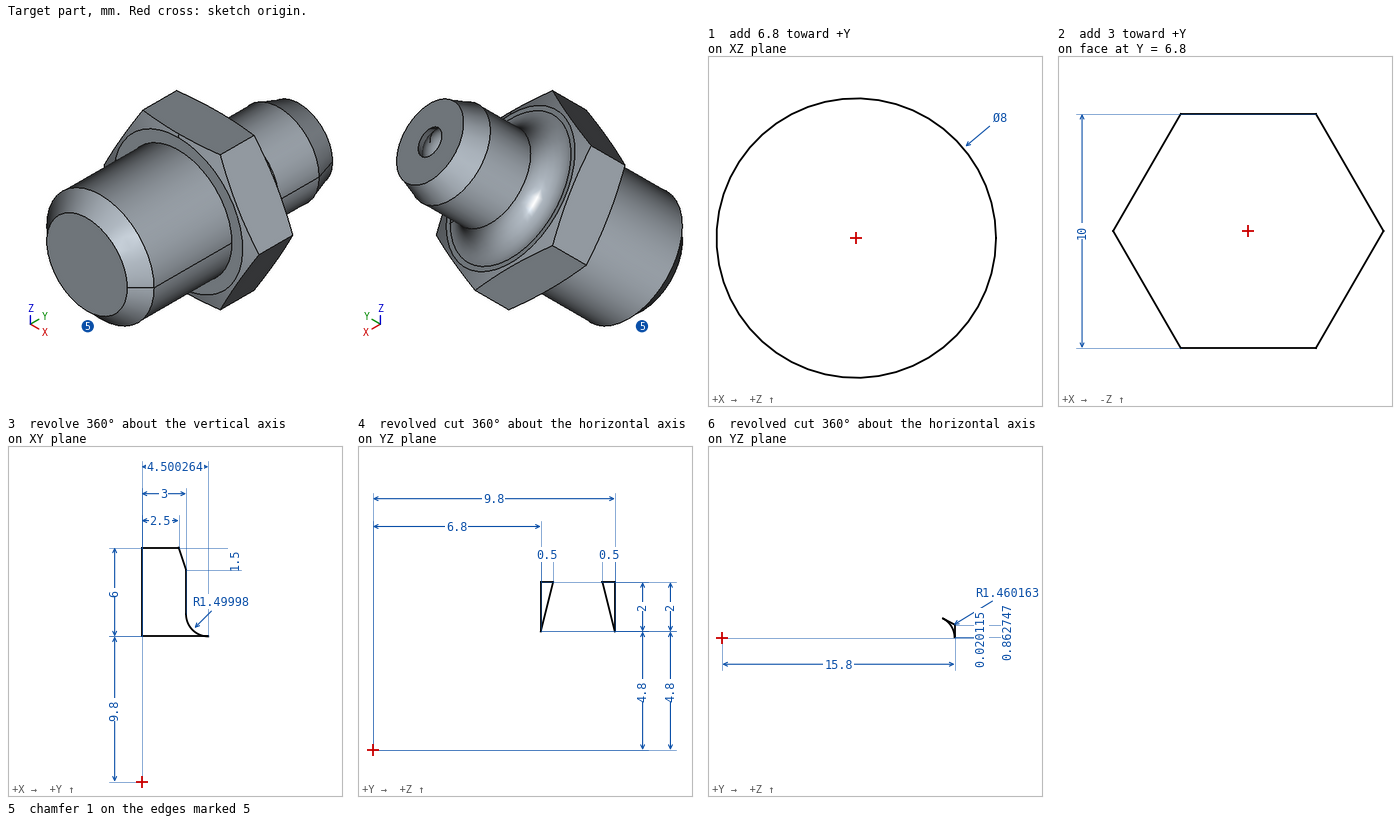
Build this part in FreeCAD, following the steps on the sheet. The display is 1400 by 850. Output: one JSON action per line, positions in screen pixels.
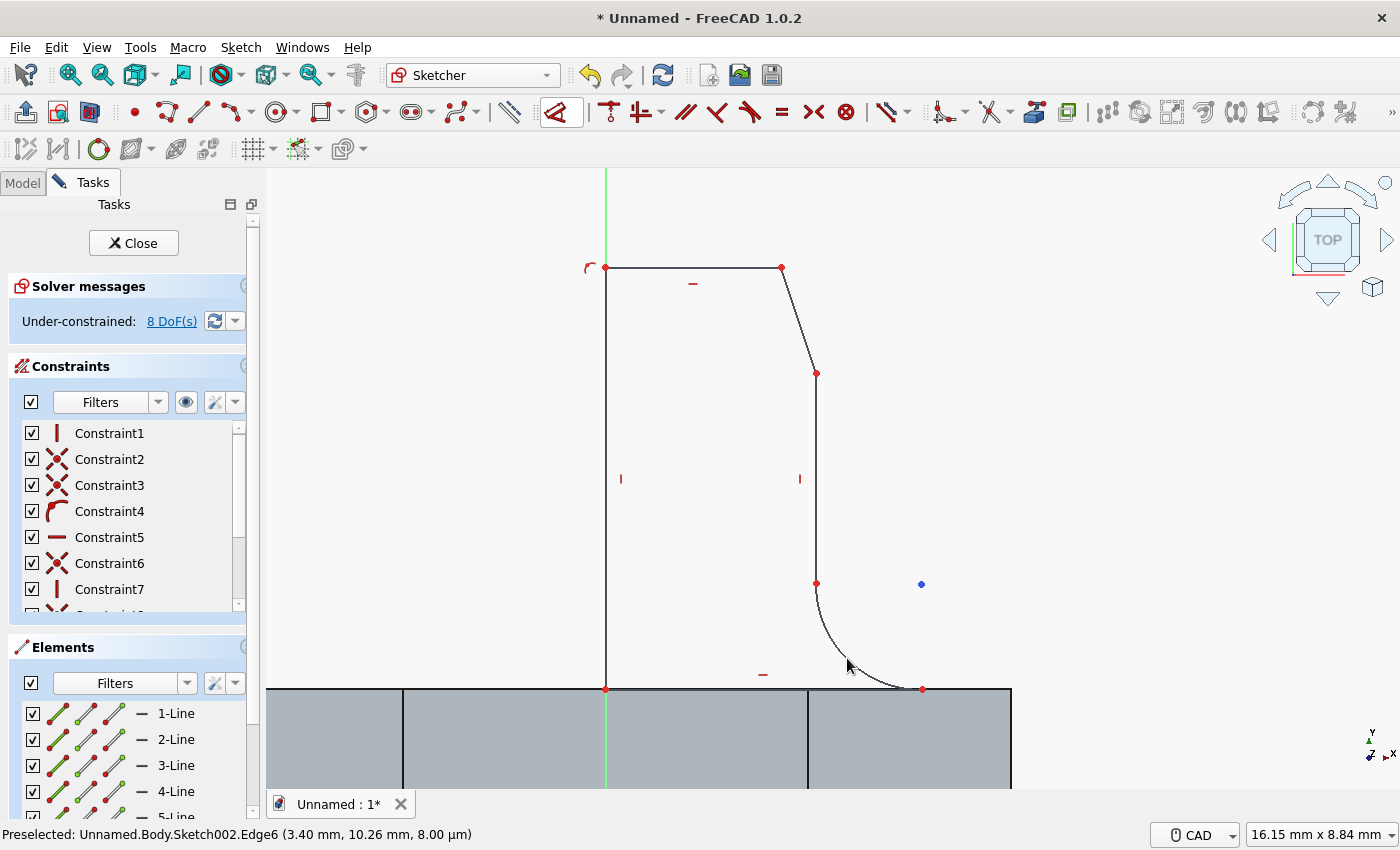
{"action": "left_click", "coordinate": [816, 521]}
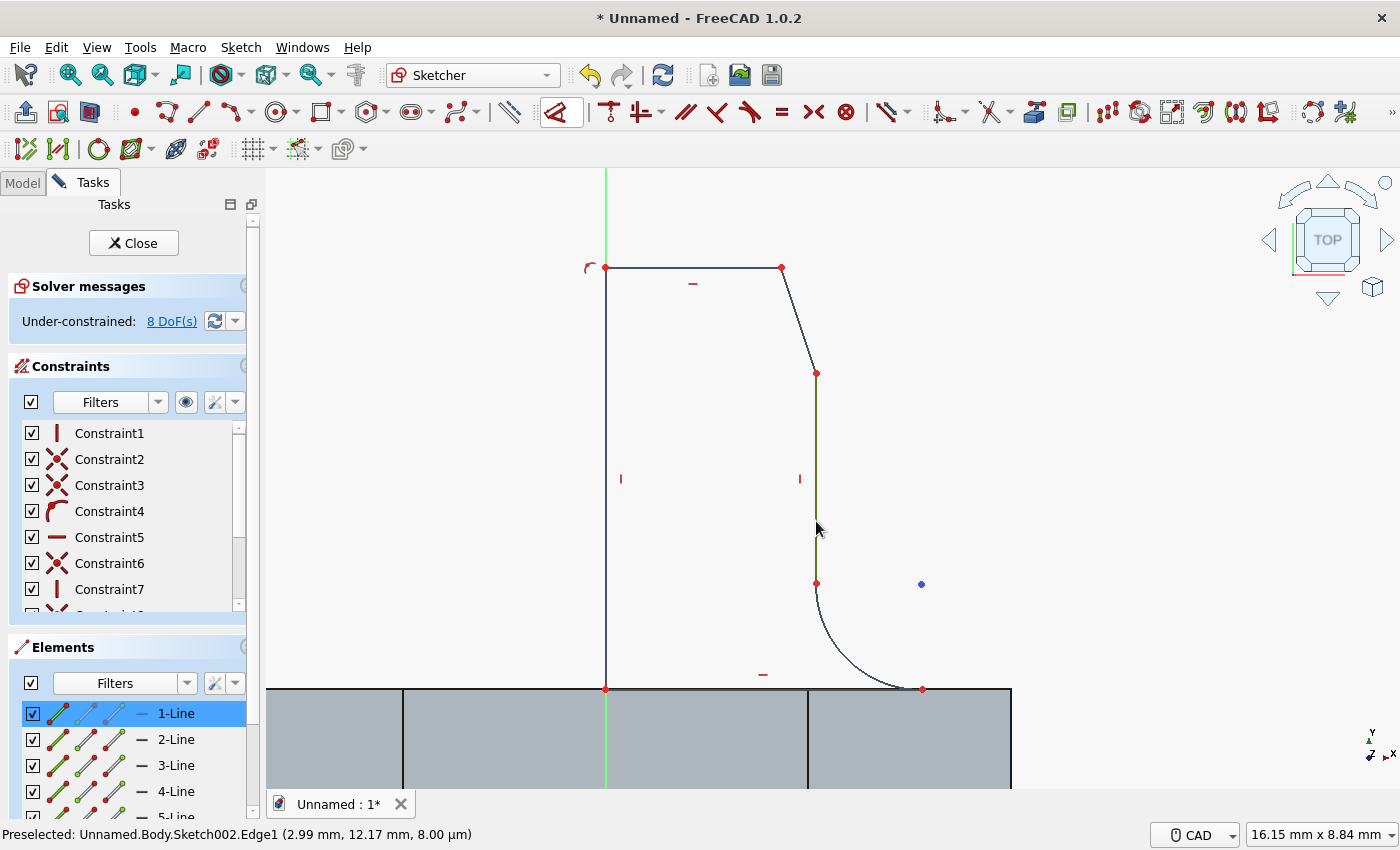
{"action": "left_click", "coordinate": [828, 632]}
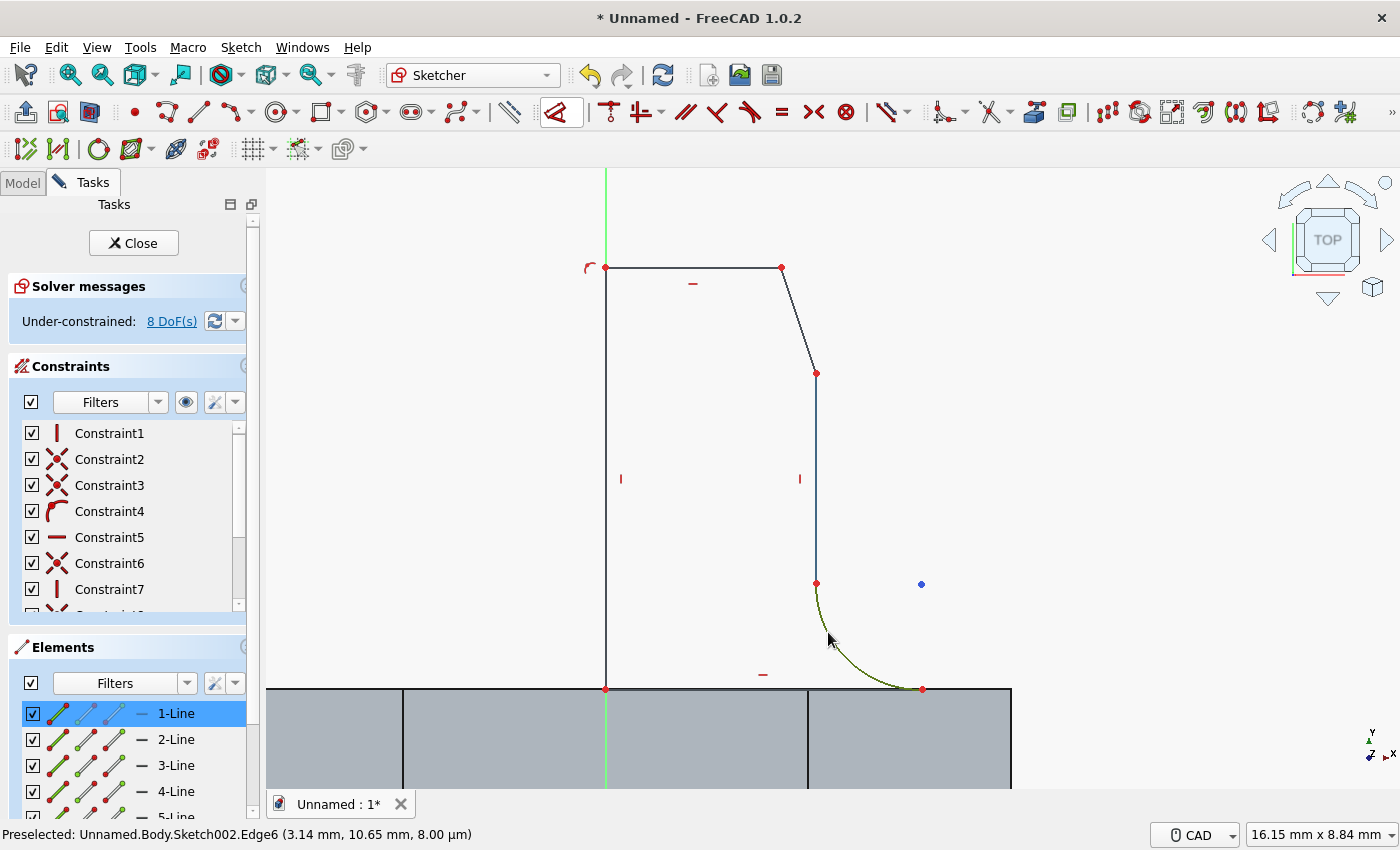
{"action": "key", "text": "t"}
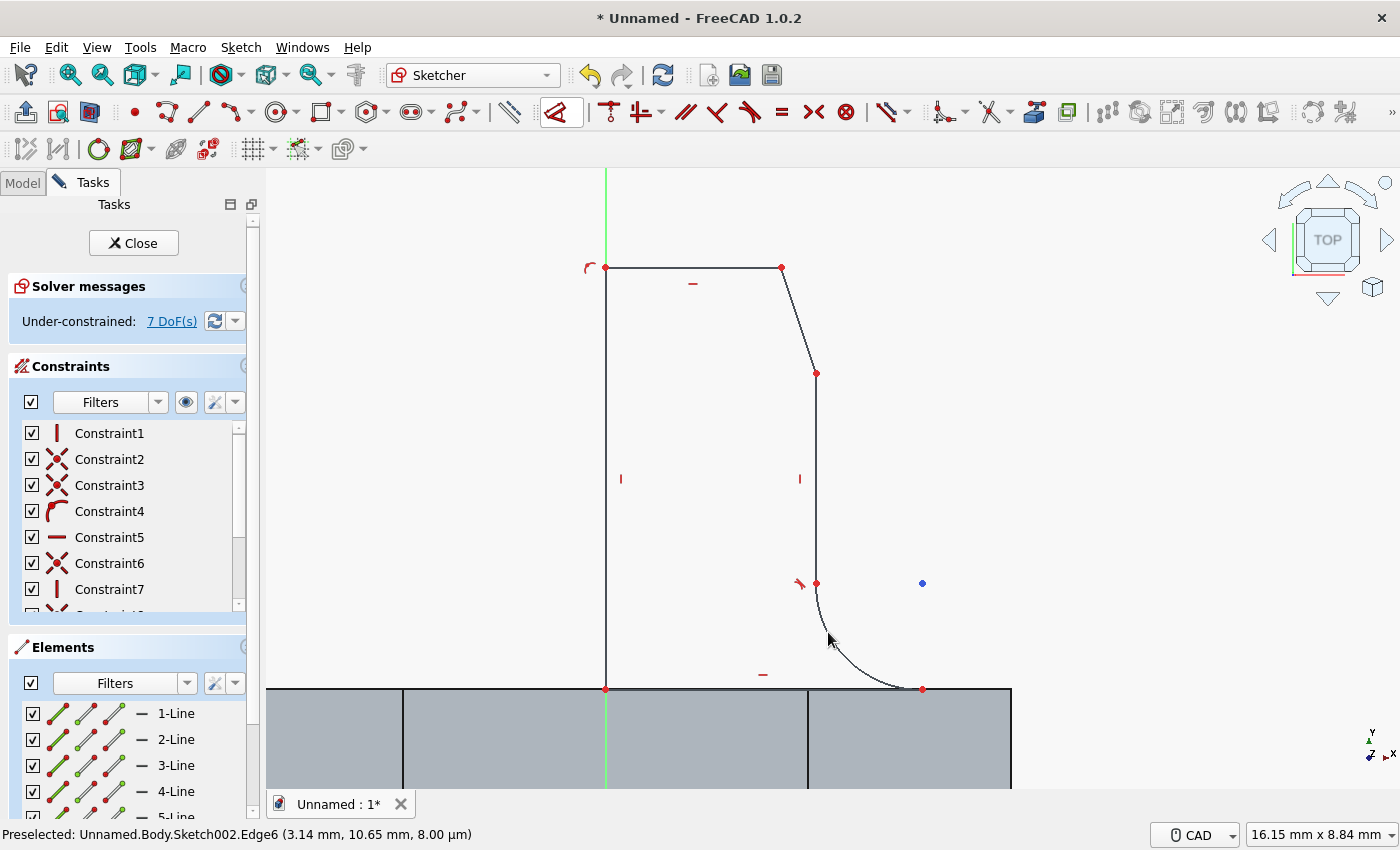
{"action": "left_click", "coordinate": [828, 632]}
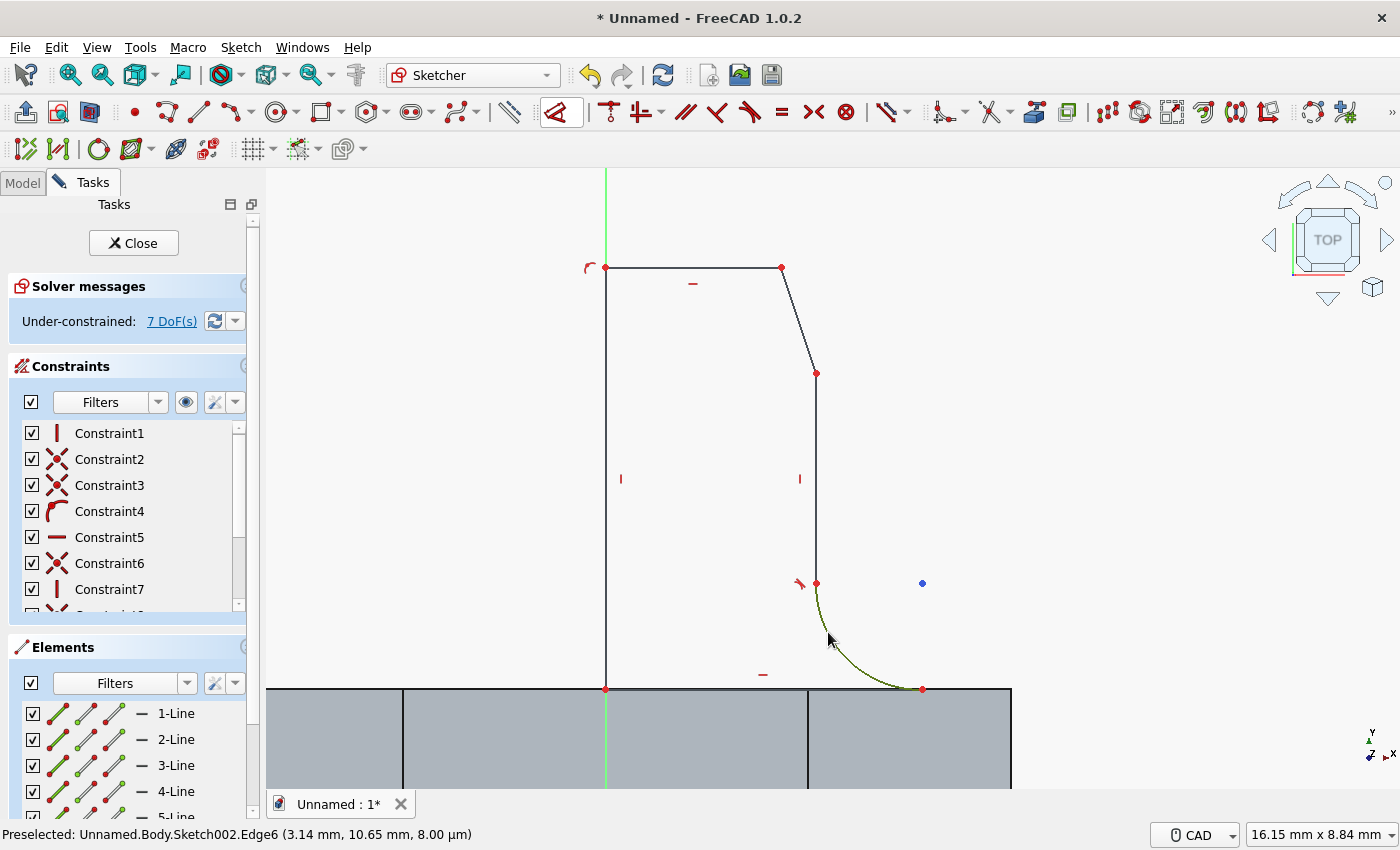
{"action": "left_click", "coordinate": [578, 112]}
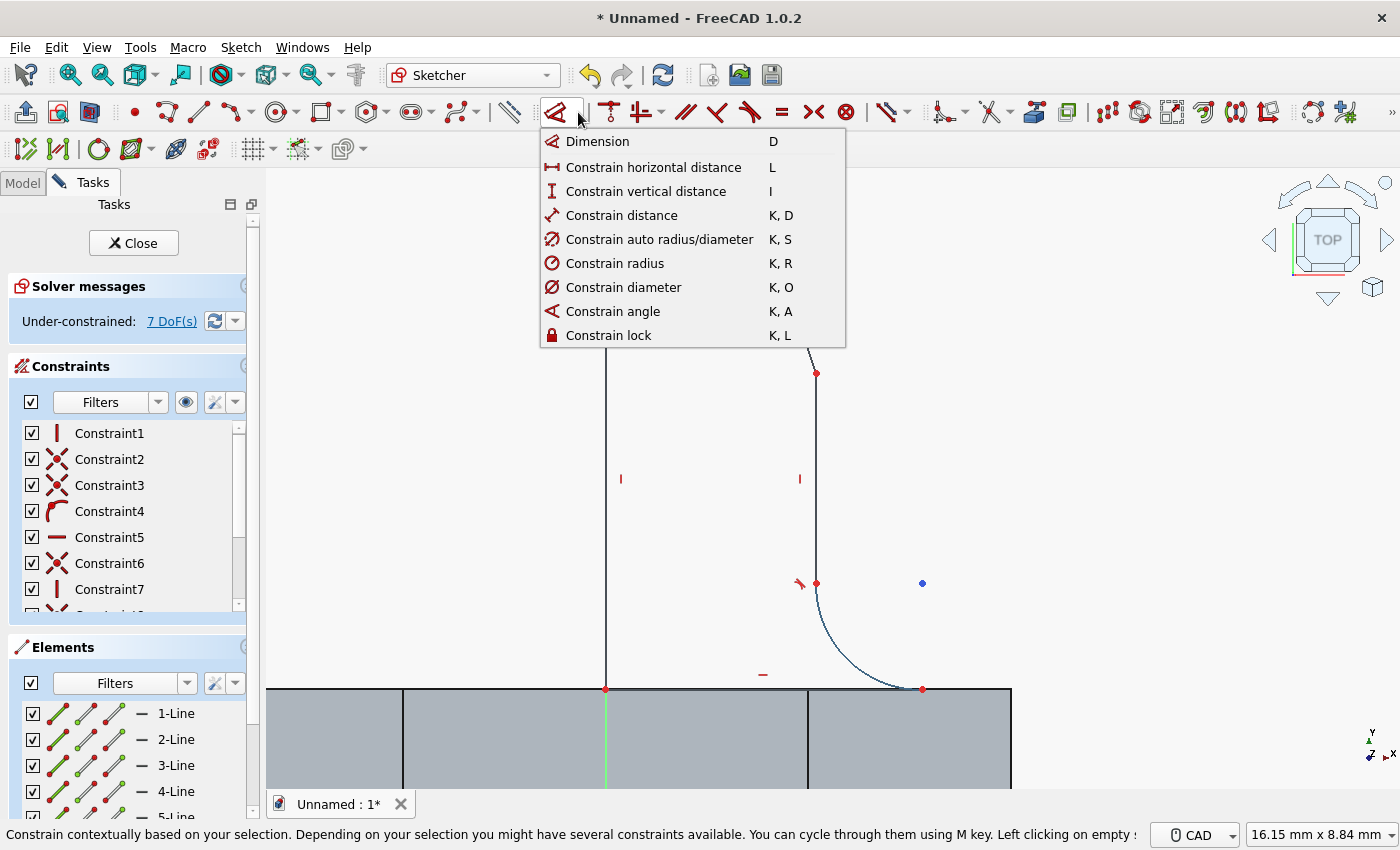
{"action": "left_click", "coordinate": [693, 263]}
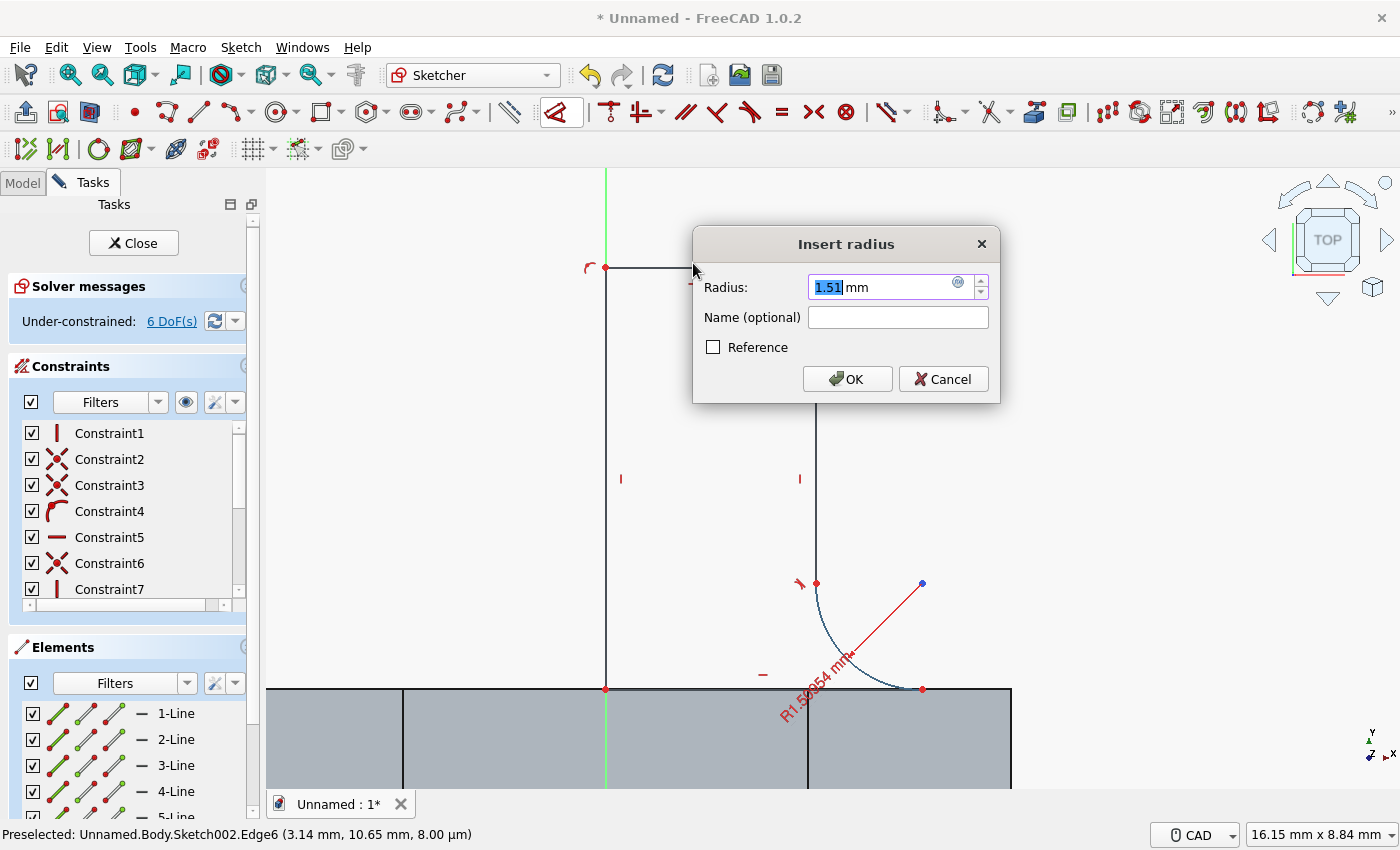
{"action": "type", "text": "1.49998"}
{"action": "key", "text": "Return"}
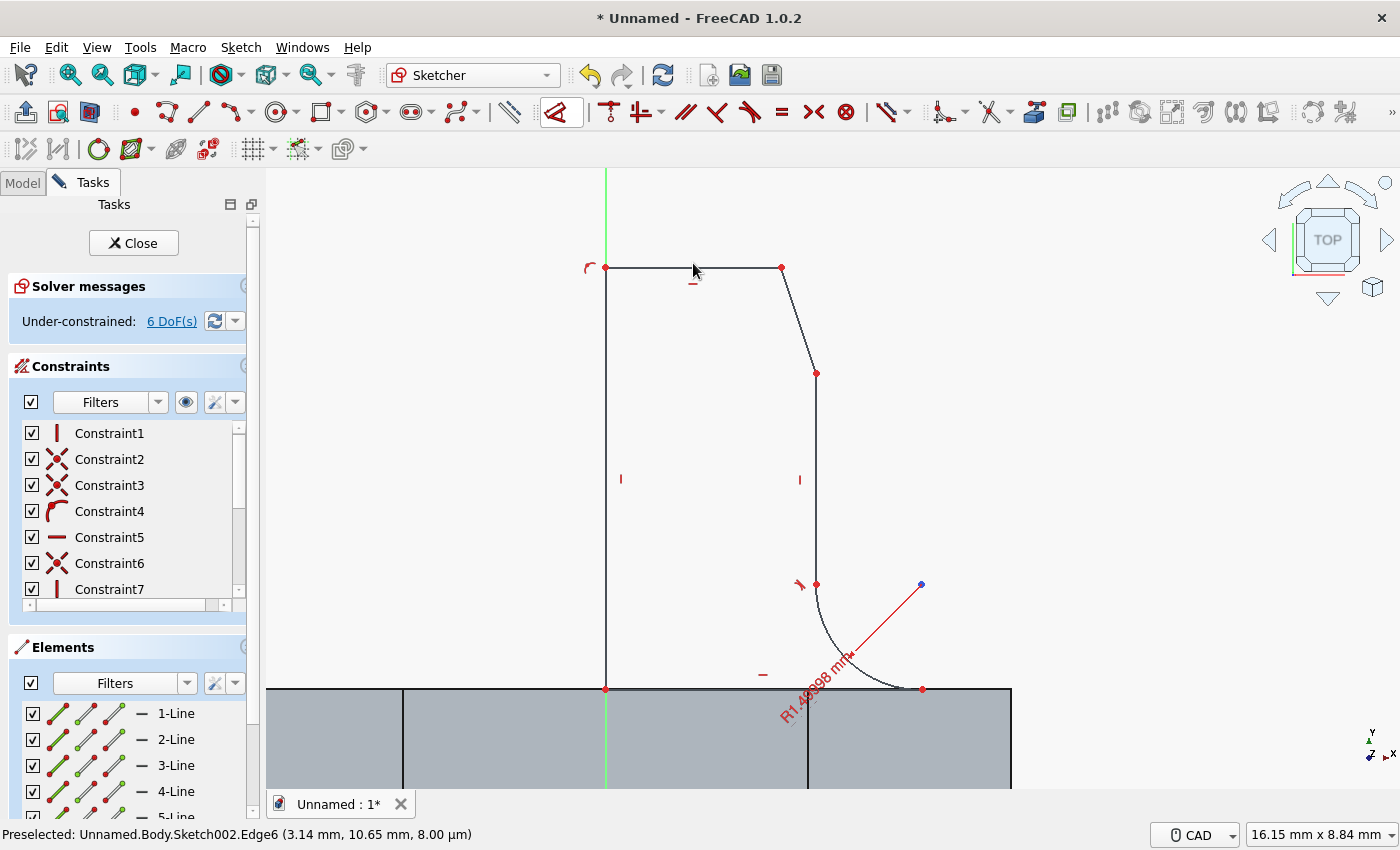
{"action": "left_click", "coordinate": [606, 395]}